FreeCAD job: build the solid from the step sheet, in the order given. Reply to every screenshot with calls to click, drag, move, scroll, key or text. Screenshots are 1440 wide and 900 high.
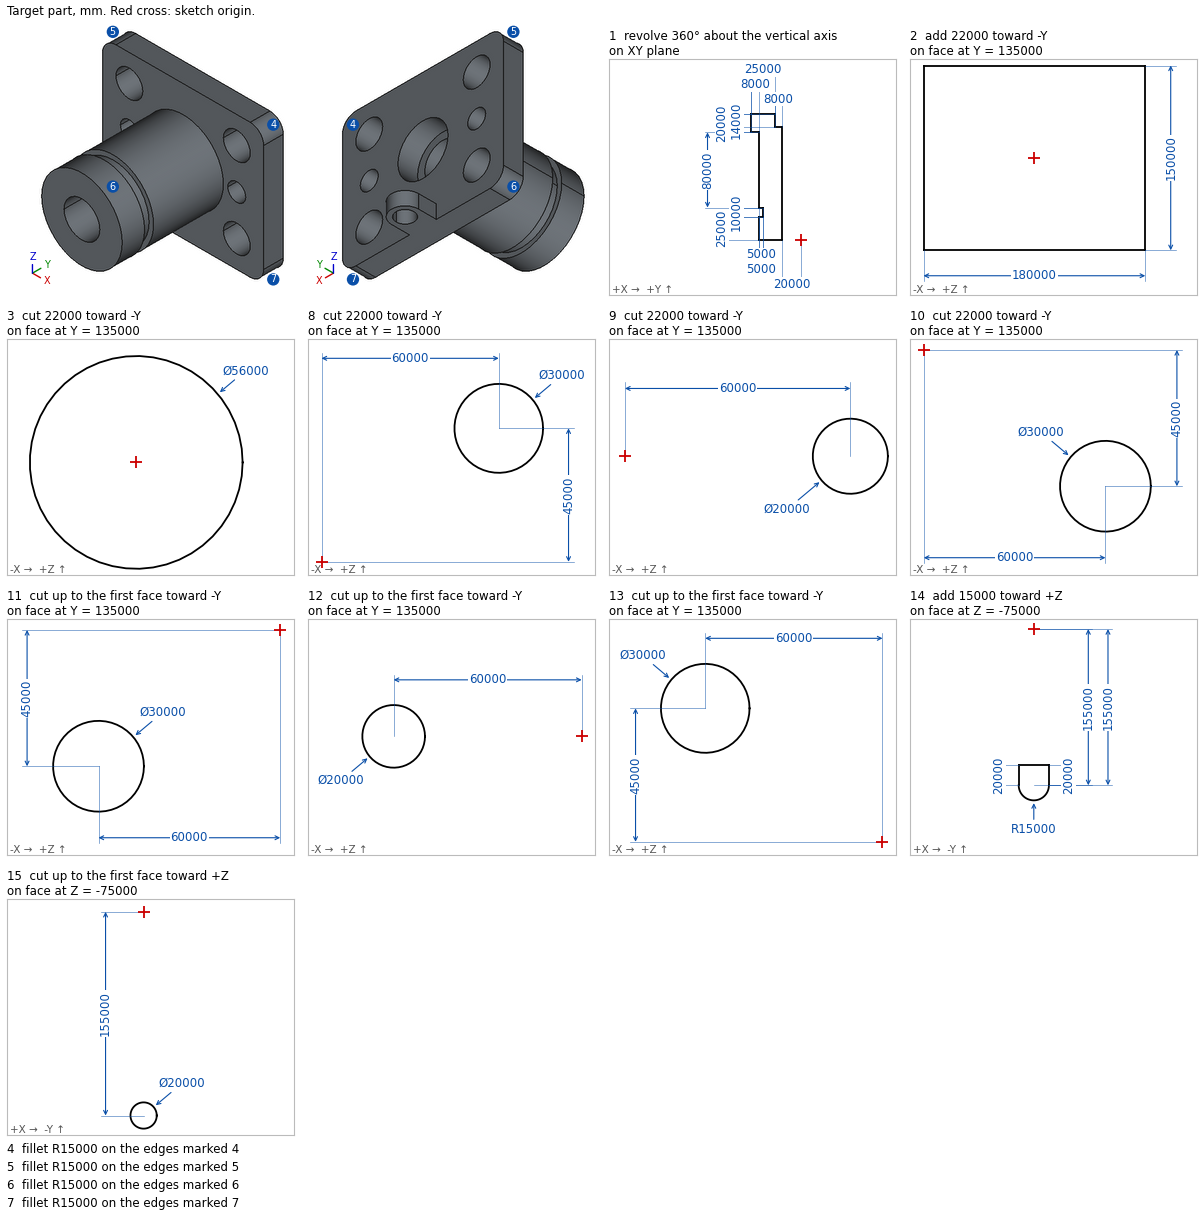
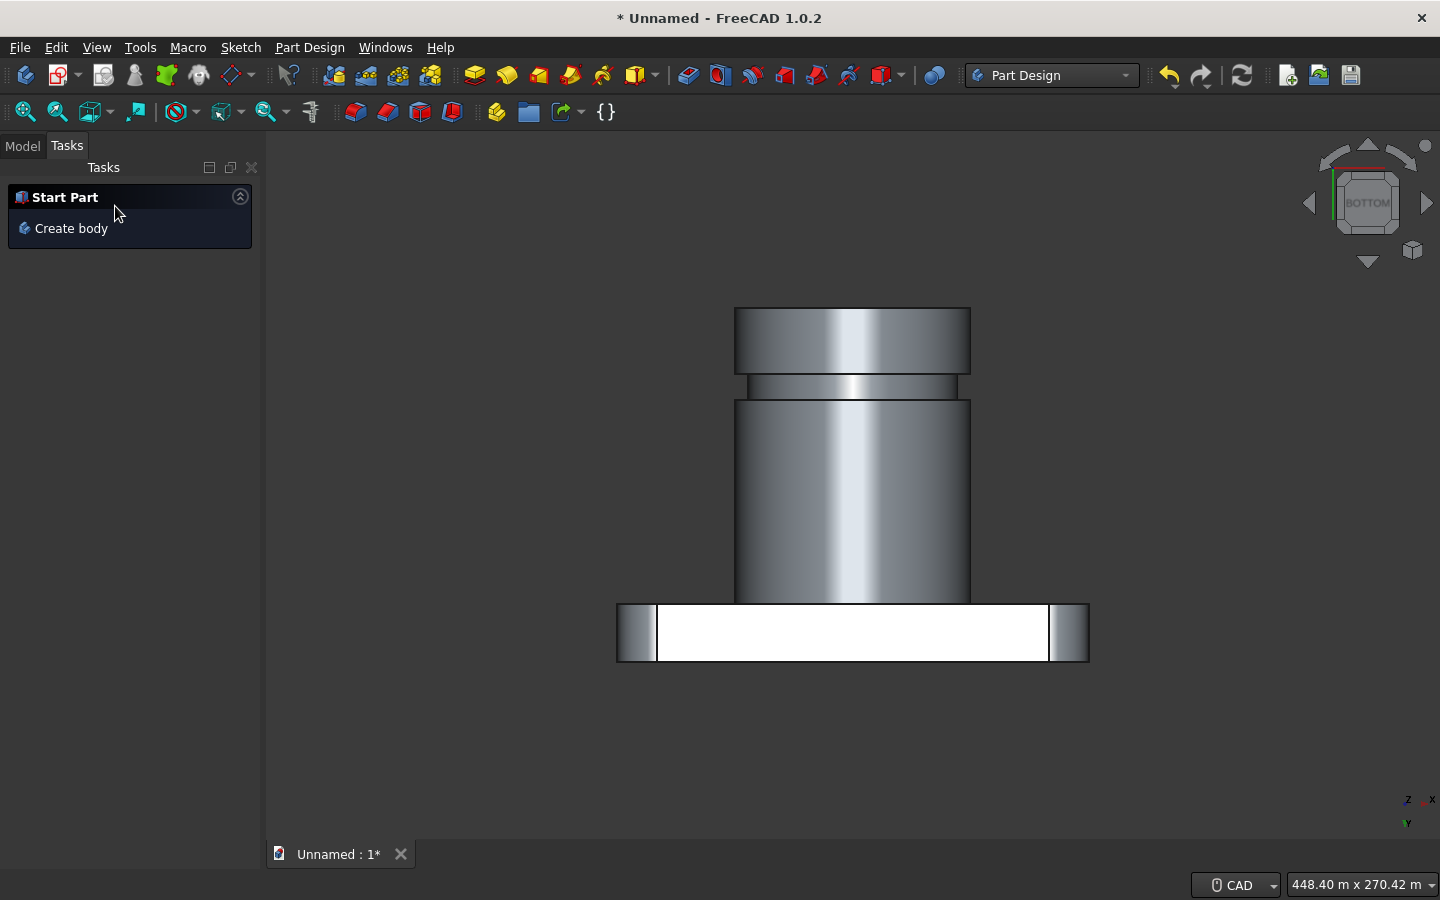
click(965, 632)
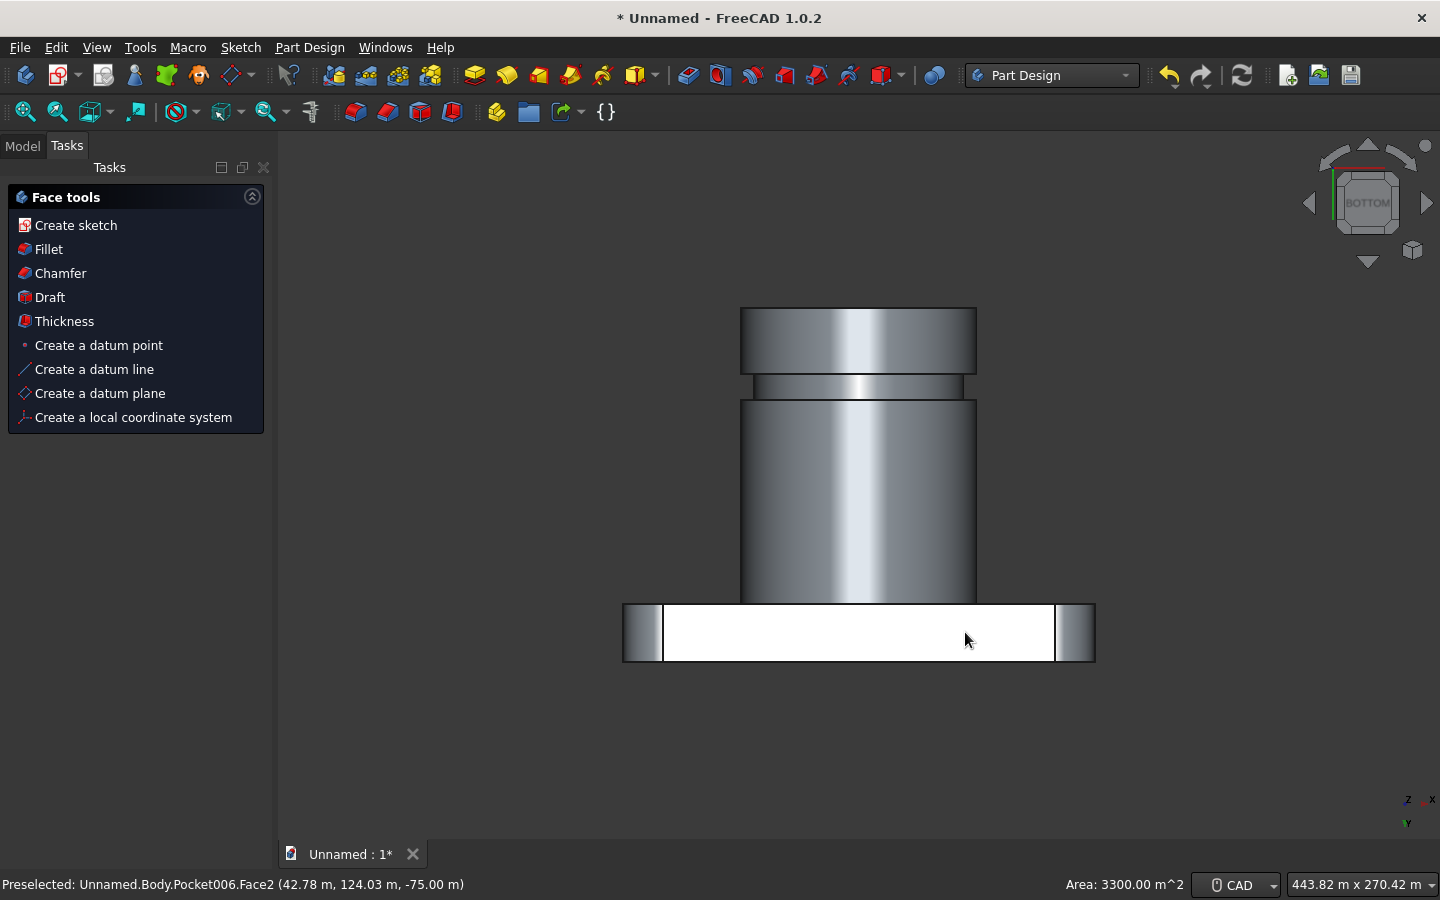
click(58, 76)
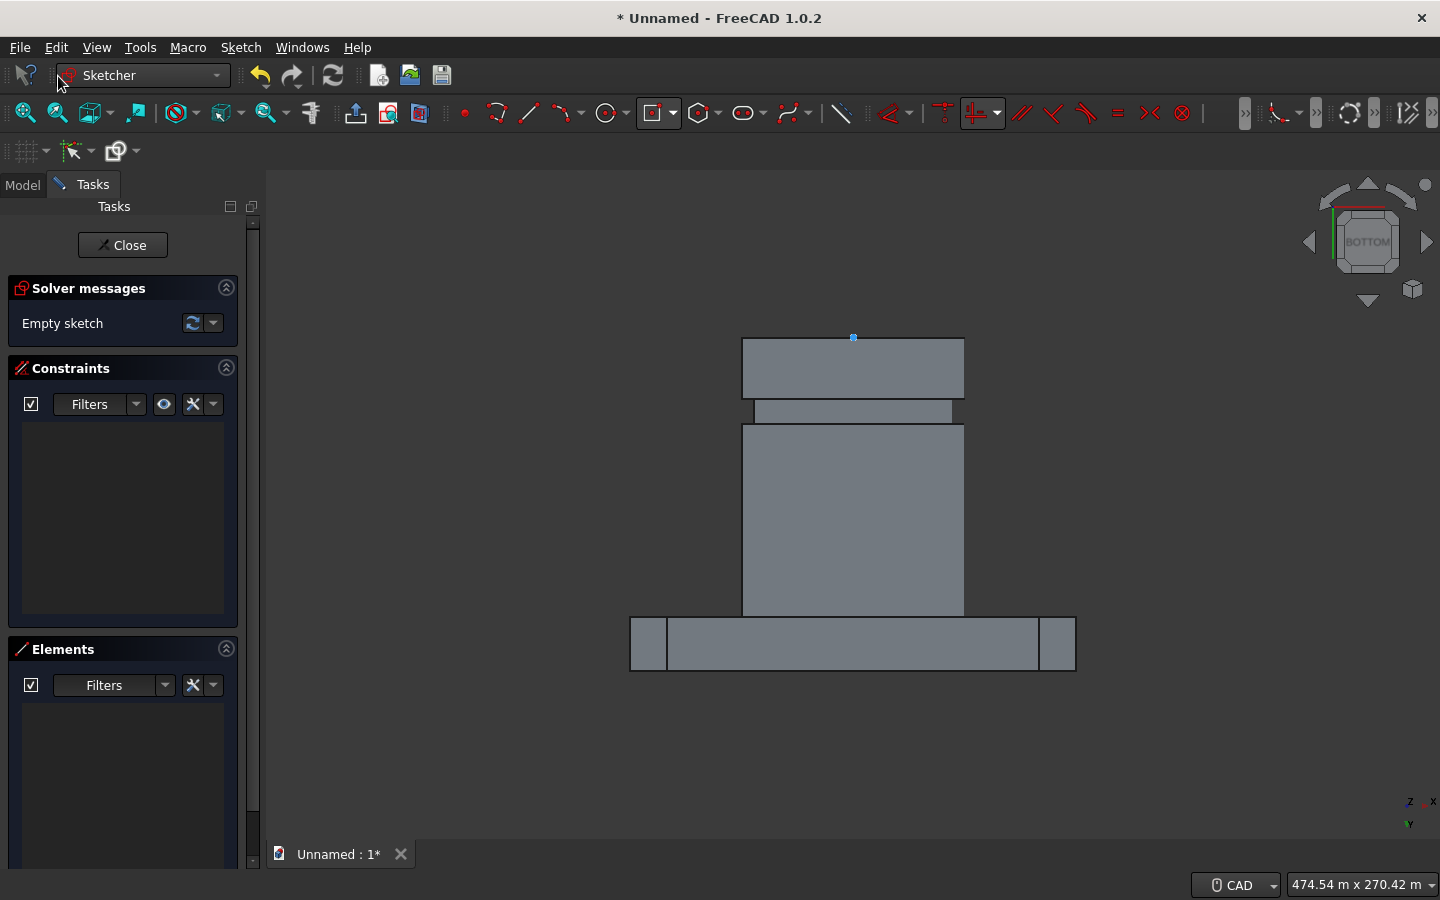
scroll(870, 768, up, 8)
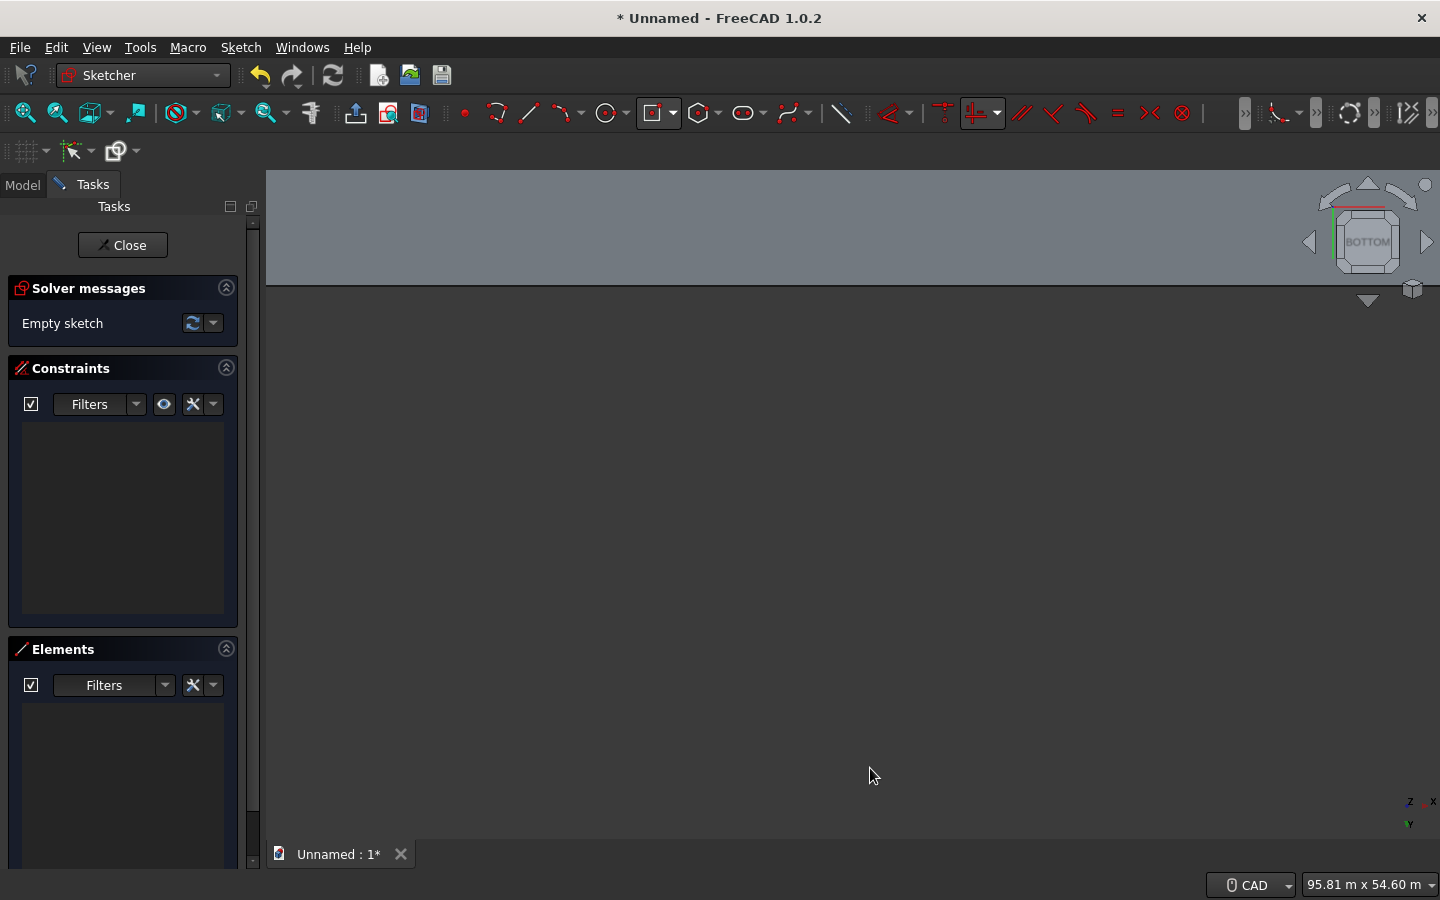
click(498, 114)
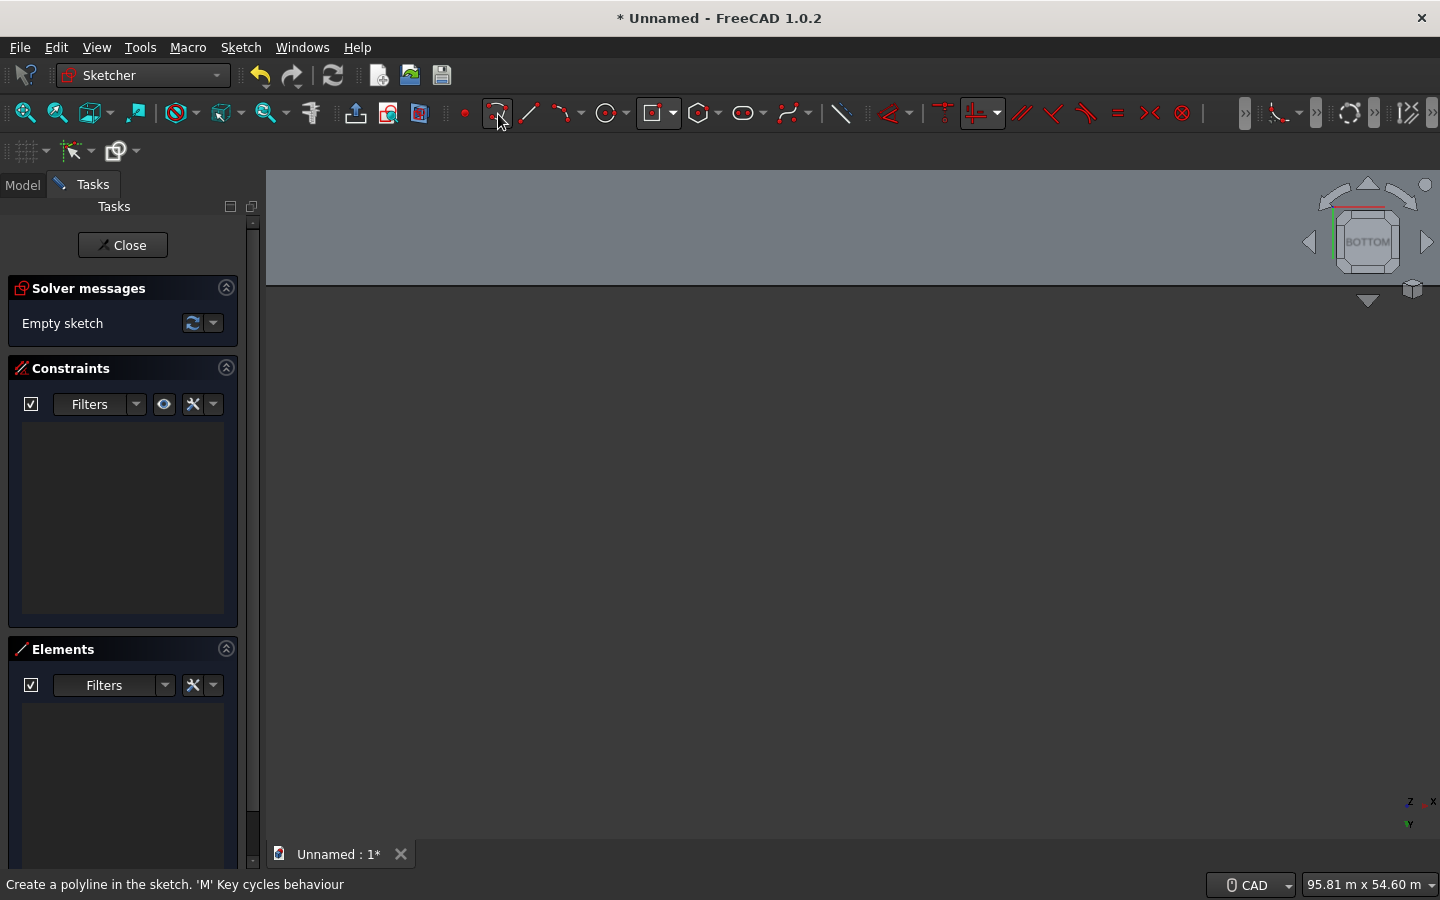
click(968, 532)
click(968, 286)
click(600, 286)
click(600, 532)
right_click(600, 532)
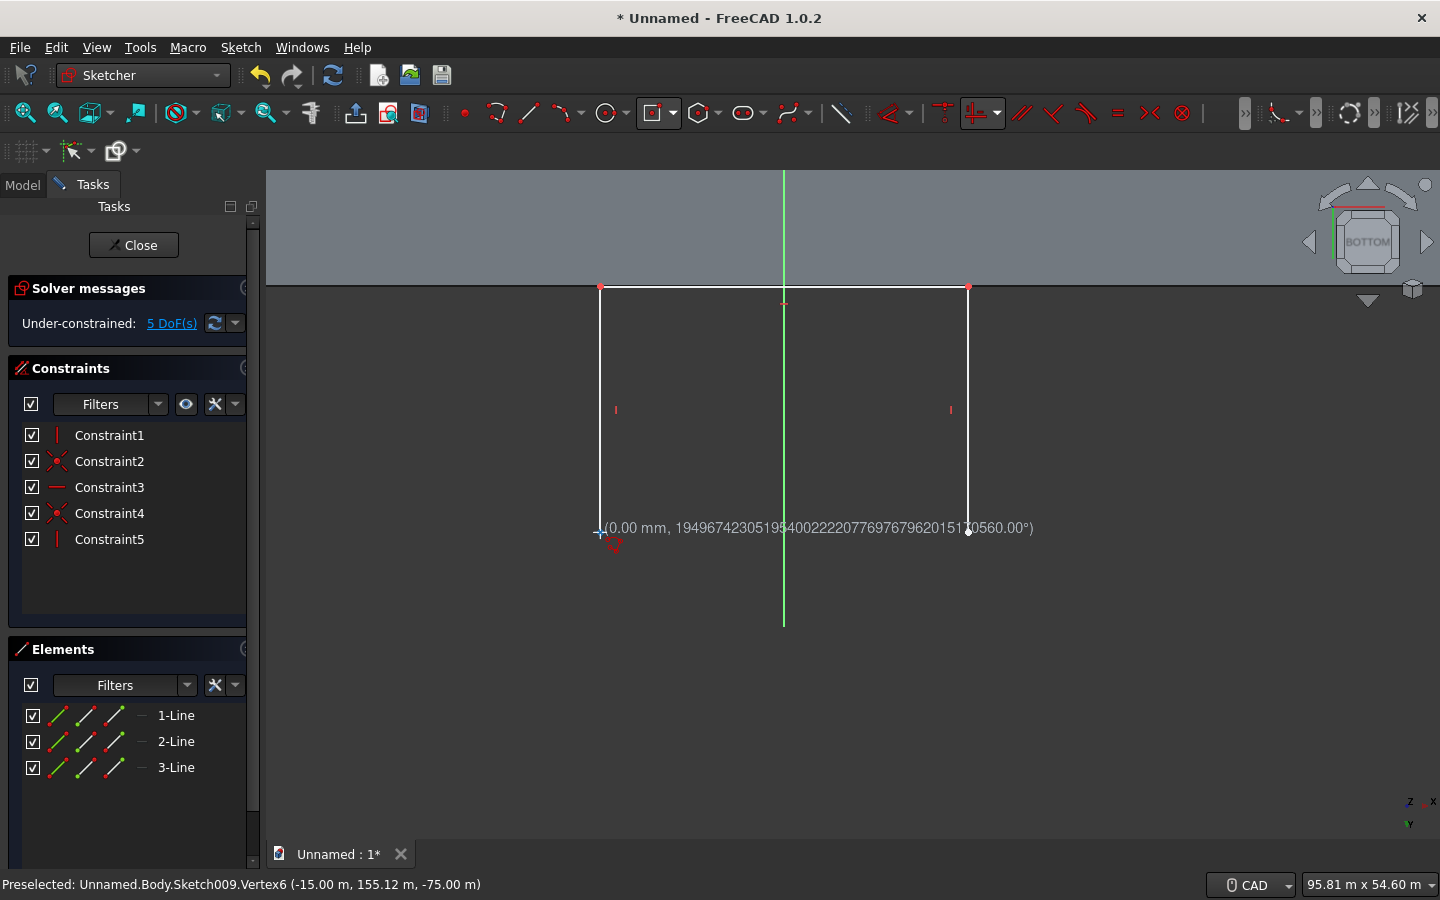
click(562, 114)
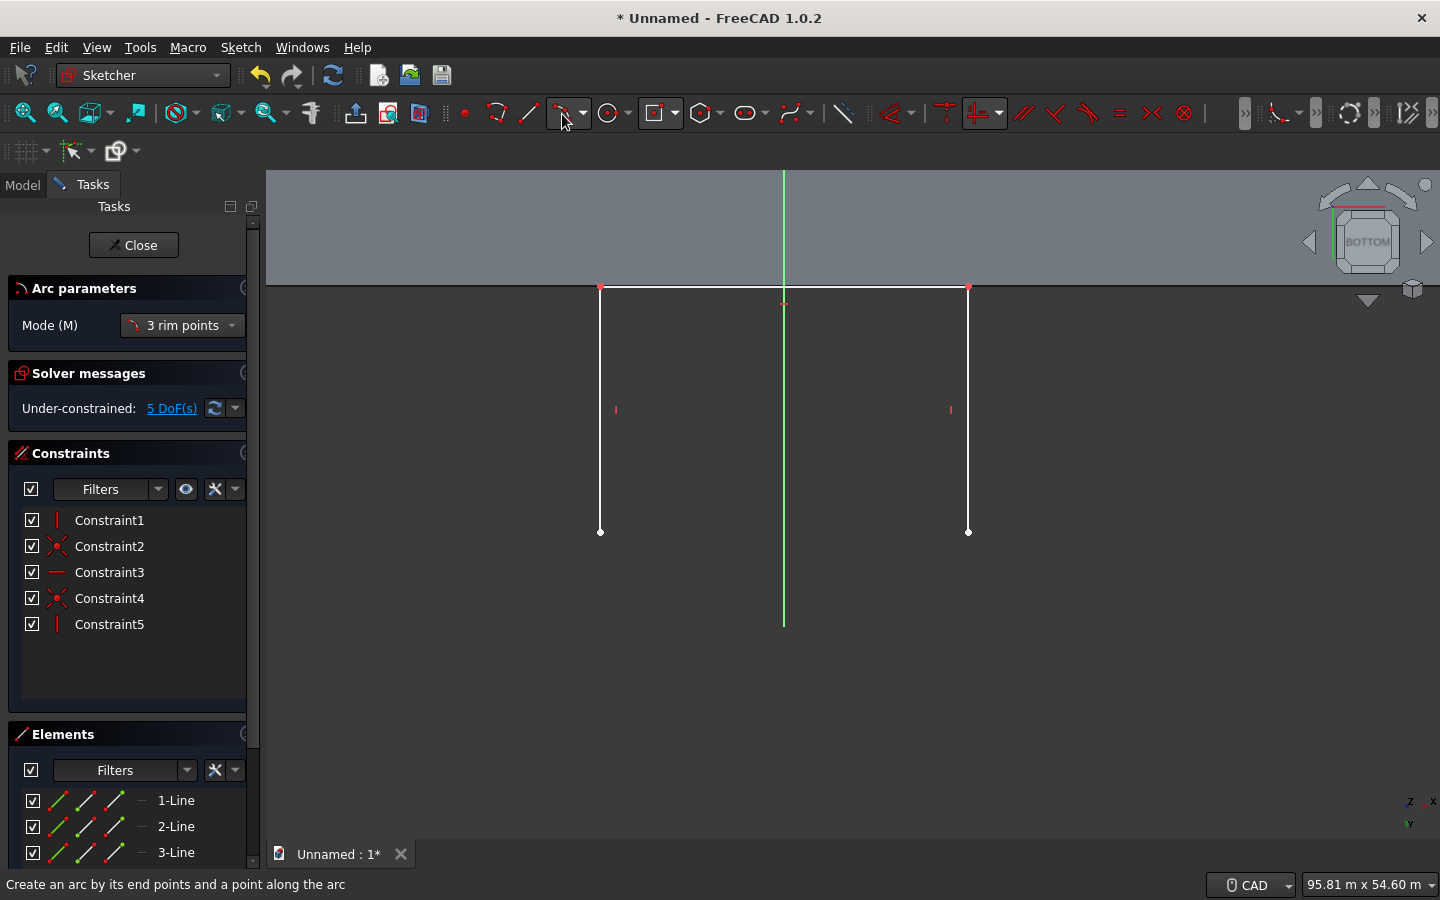
click(600, 533)
click(968, 533)
click(727, 706)
key(Escape)